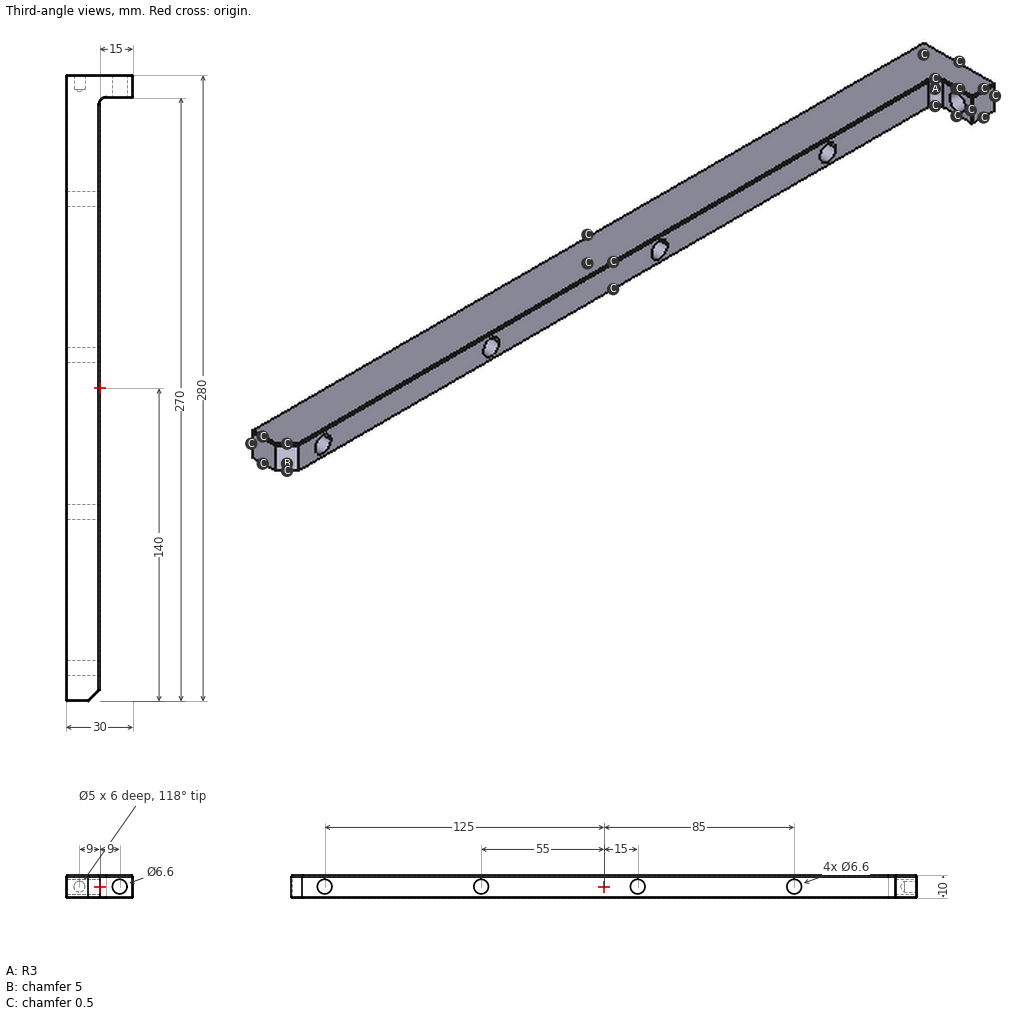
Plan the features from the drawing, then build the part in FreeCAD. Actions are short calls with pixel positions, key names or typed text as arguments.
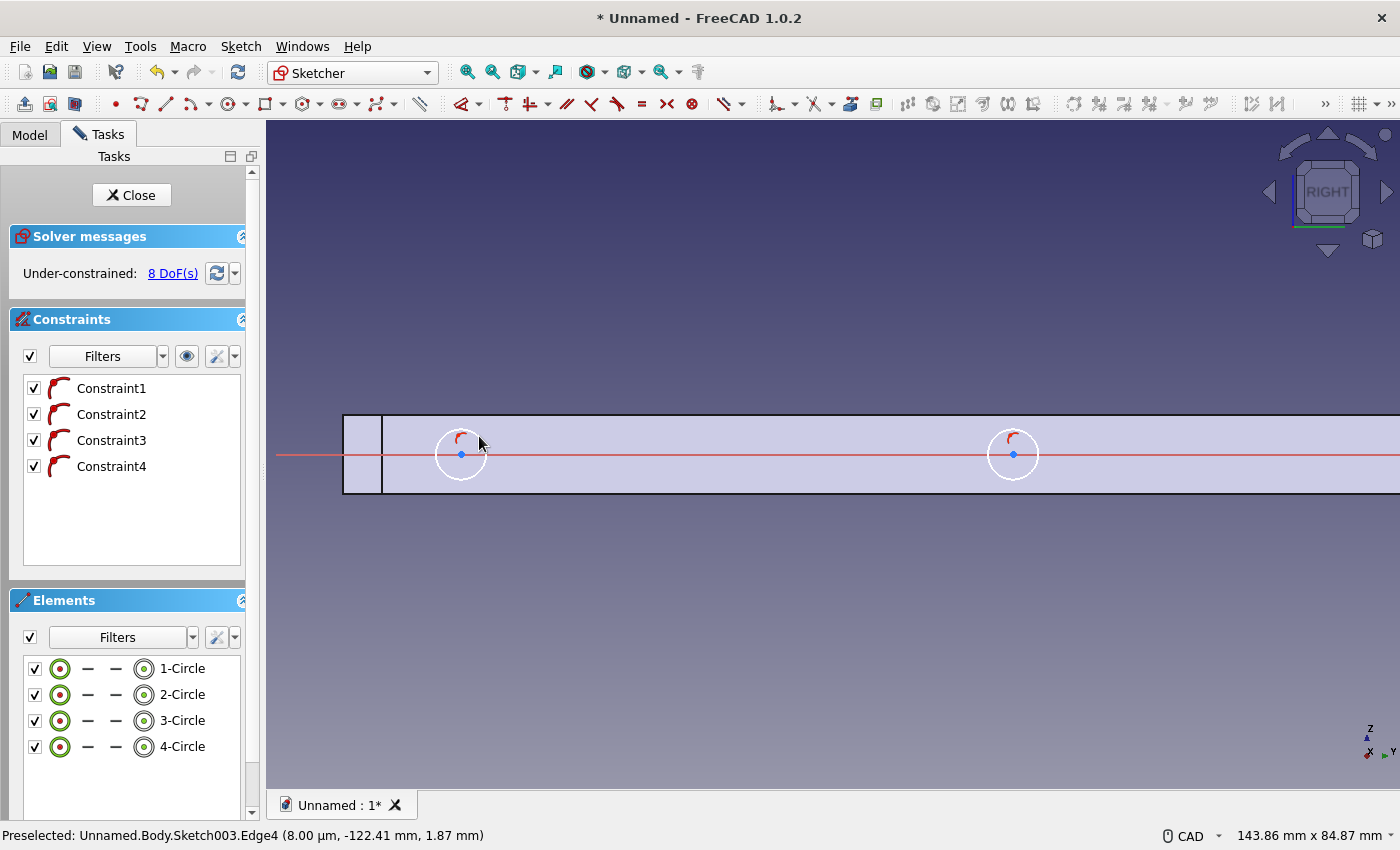
scroll(459, 455, down, 5)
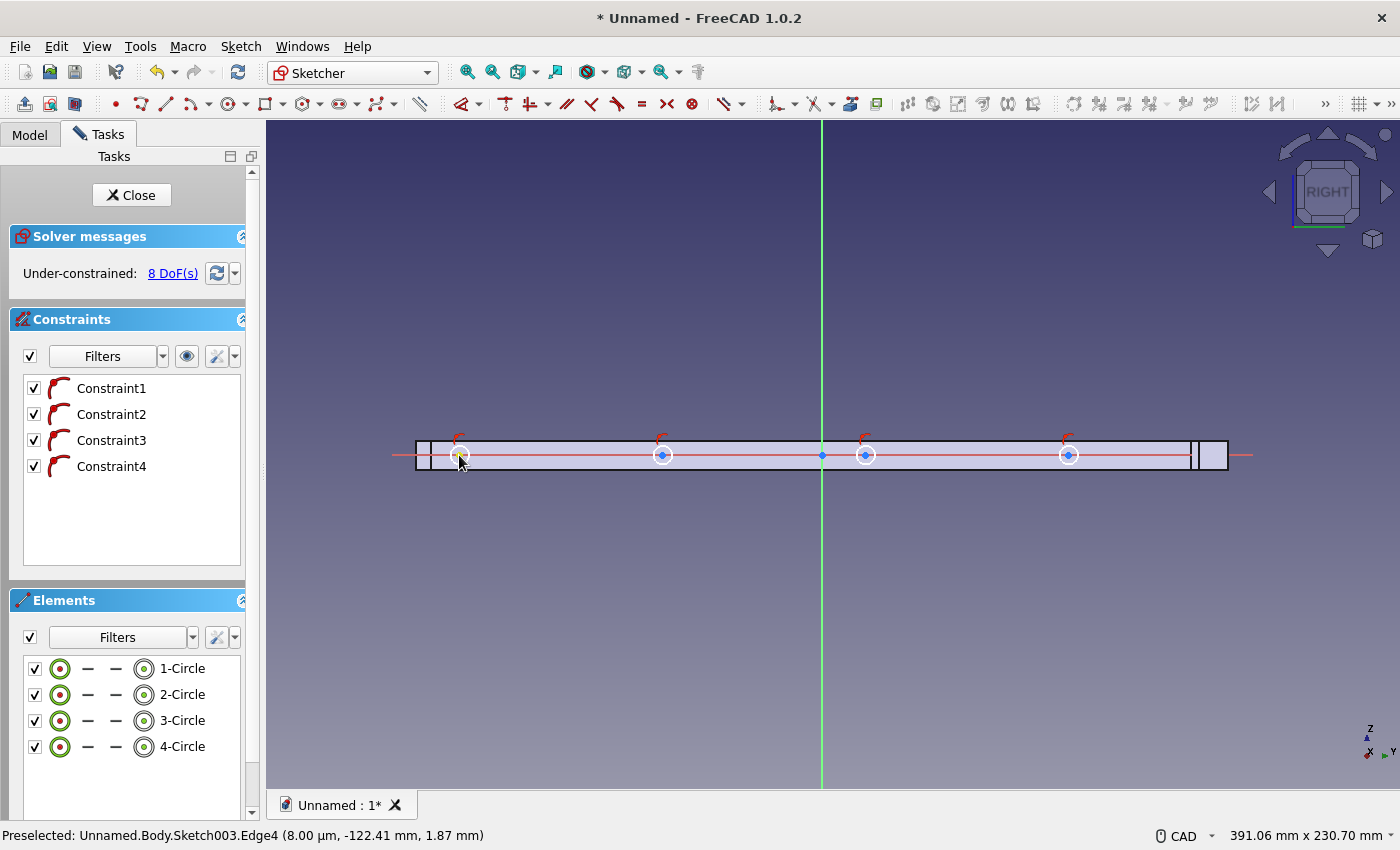
scroll(1075, 449, up, 4)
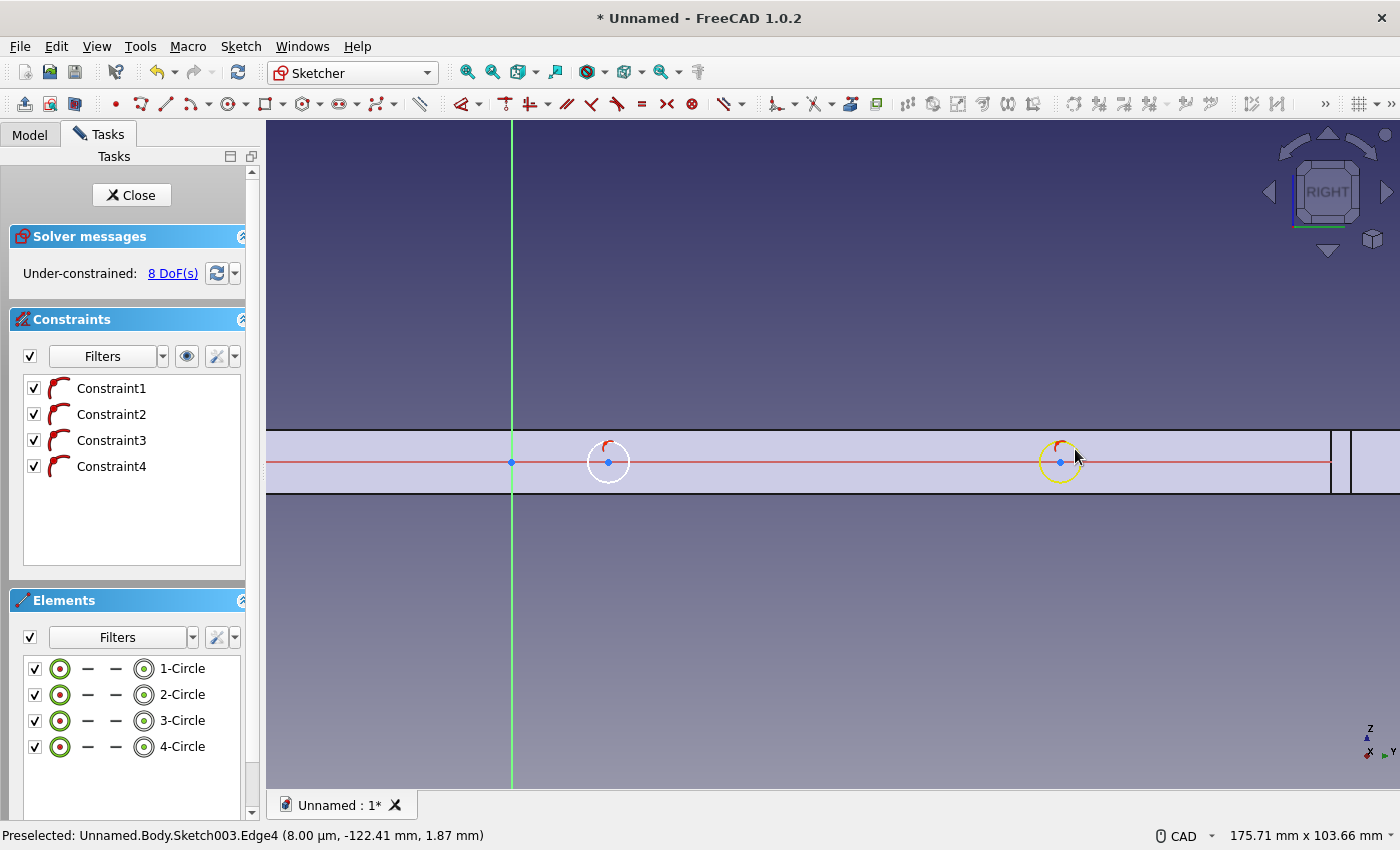
click(1075, 447)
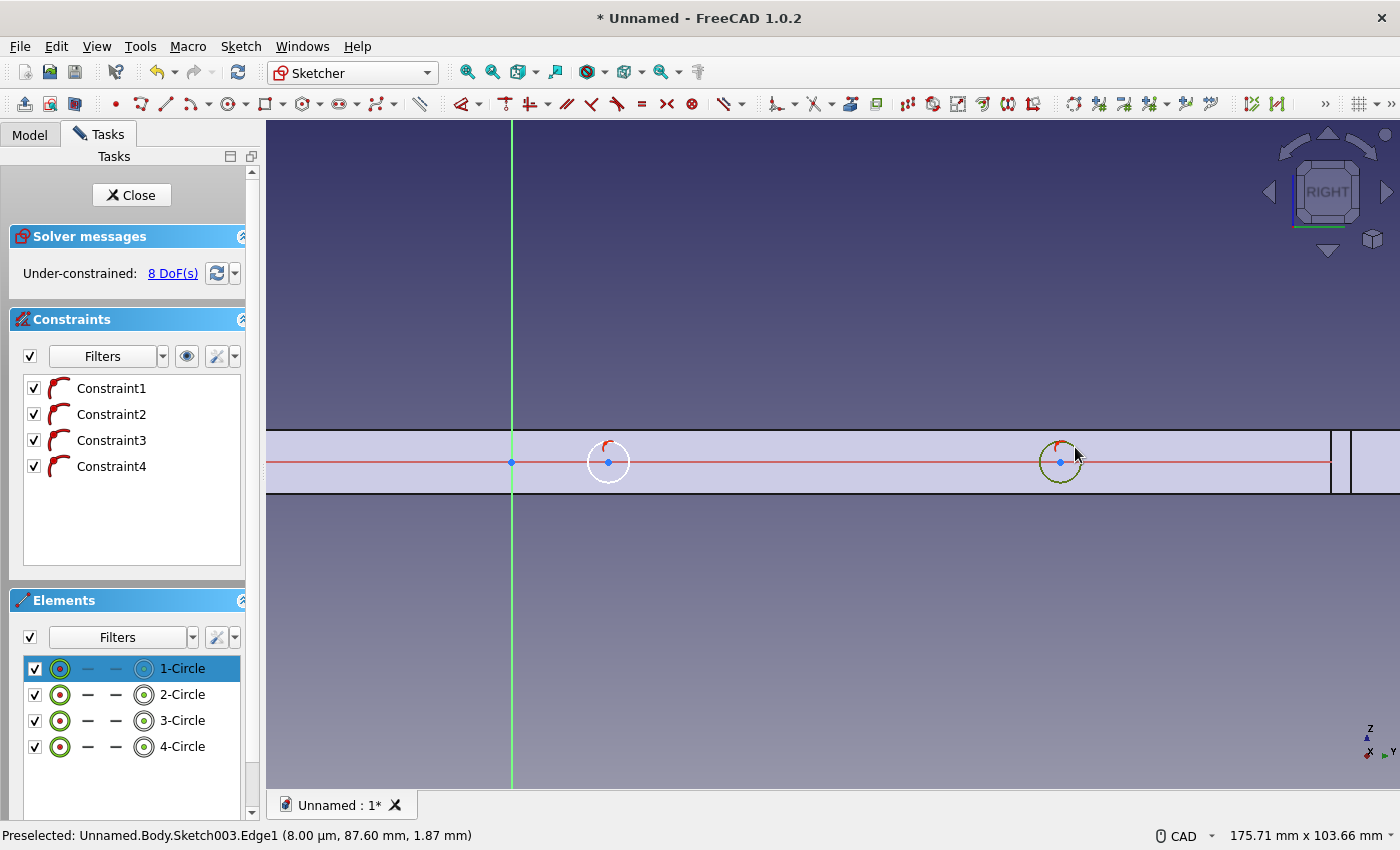
click(623, 447)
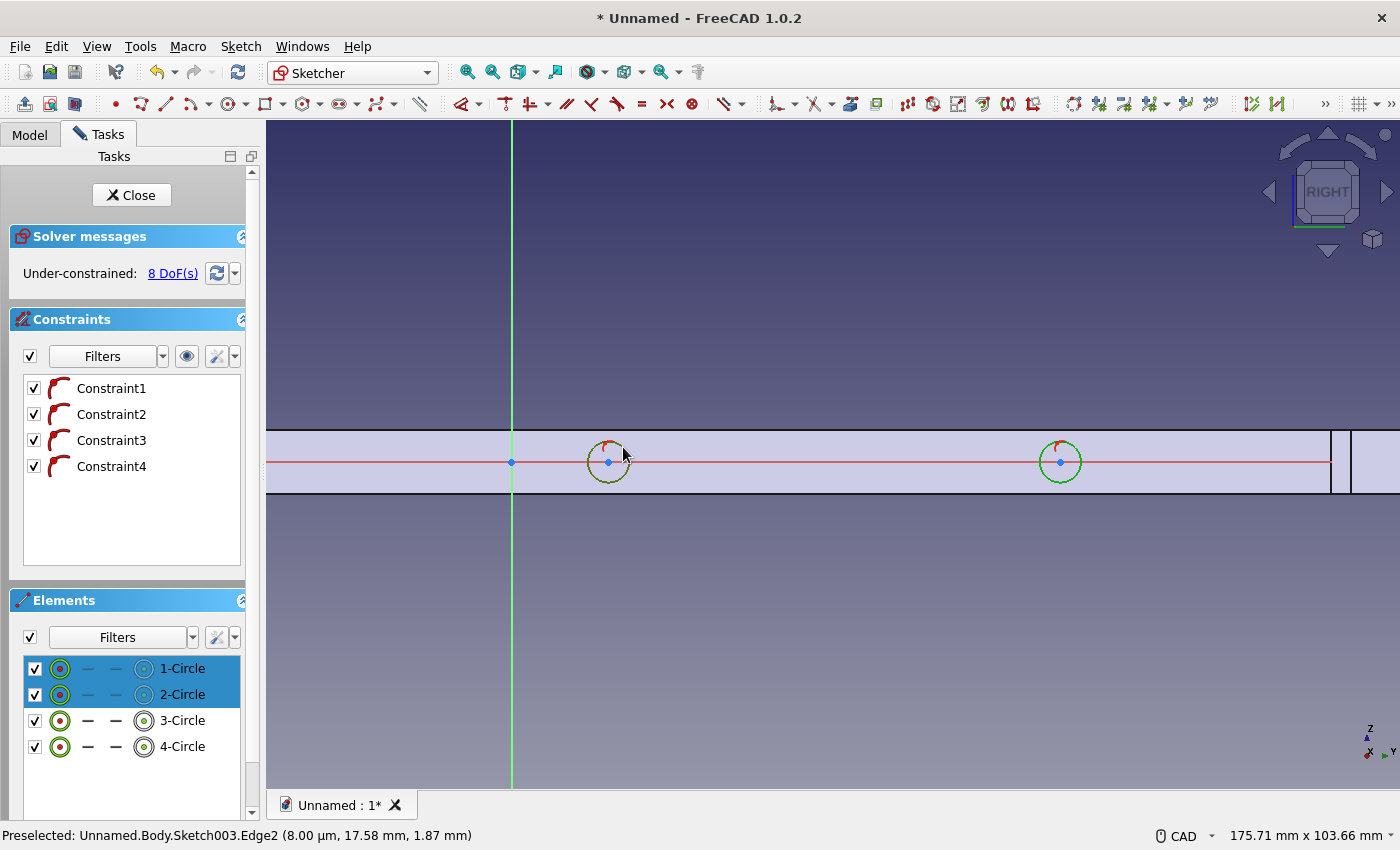
scroll(1076, 448, down, 4)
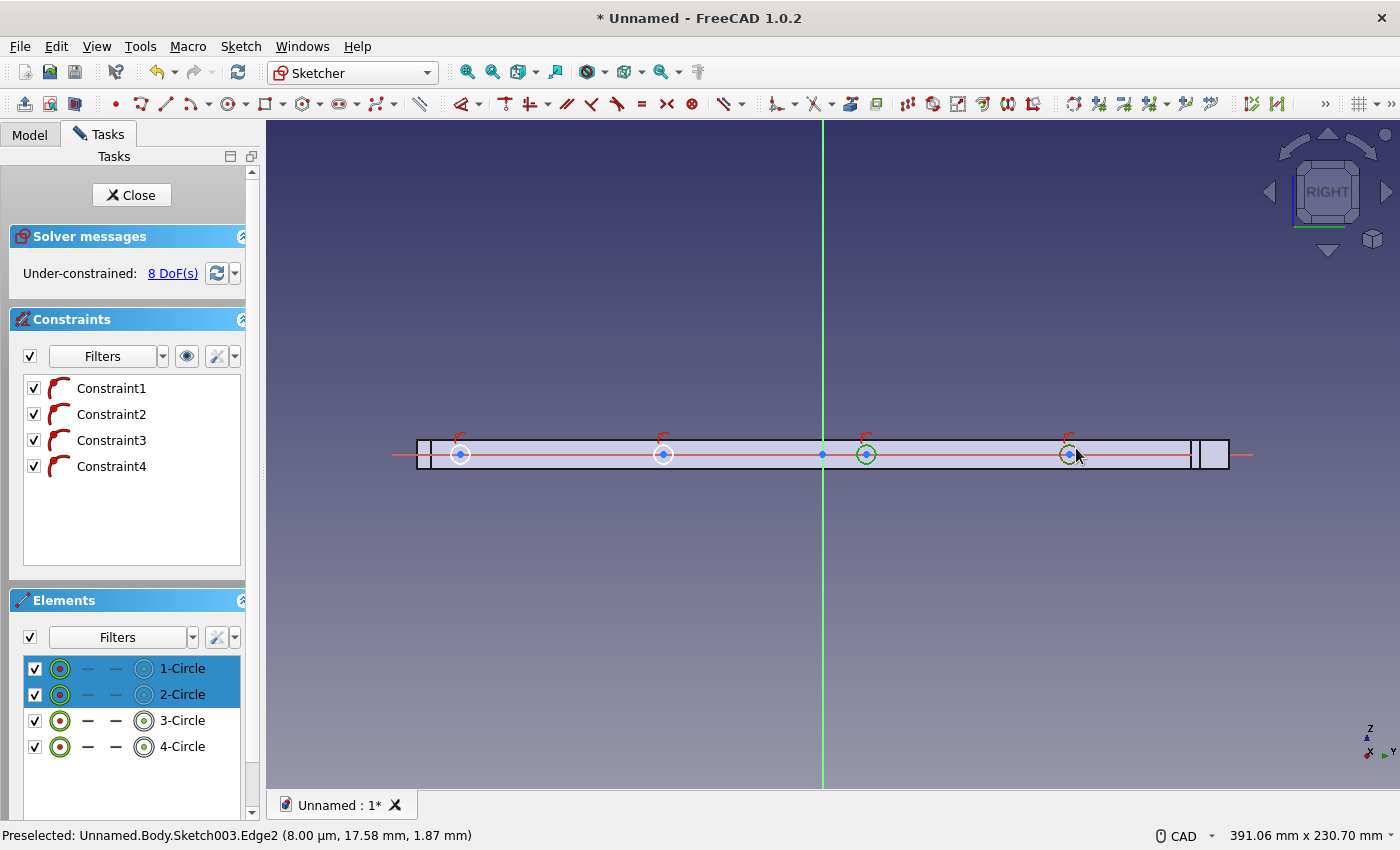
scroll(670, 448, up, 4)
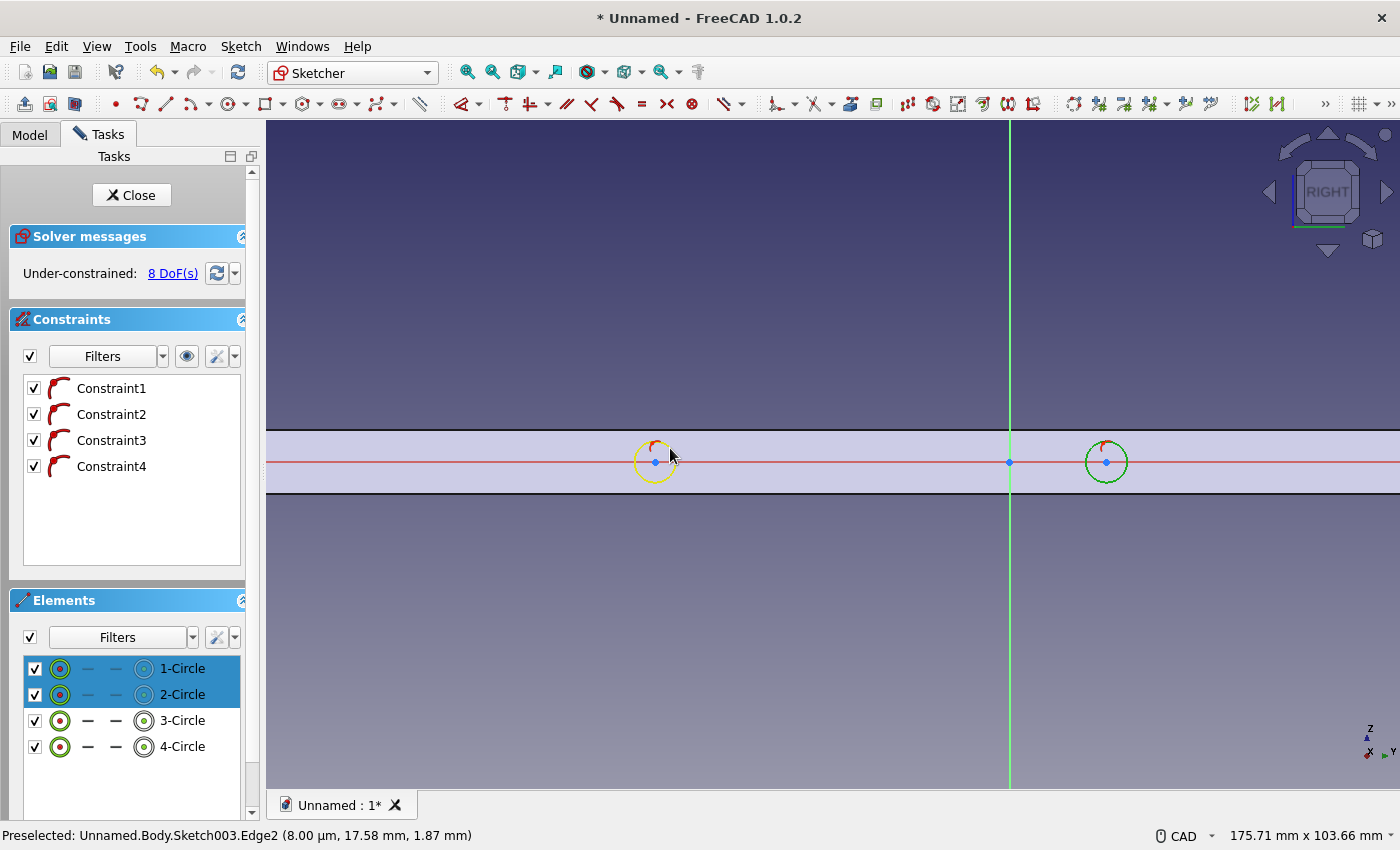
click(670, 447)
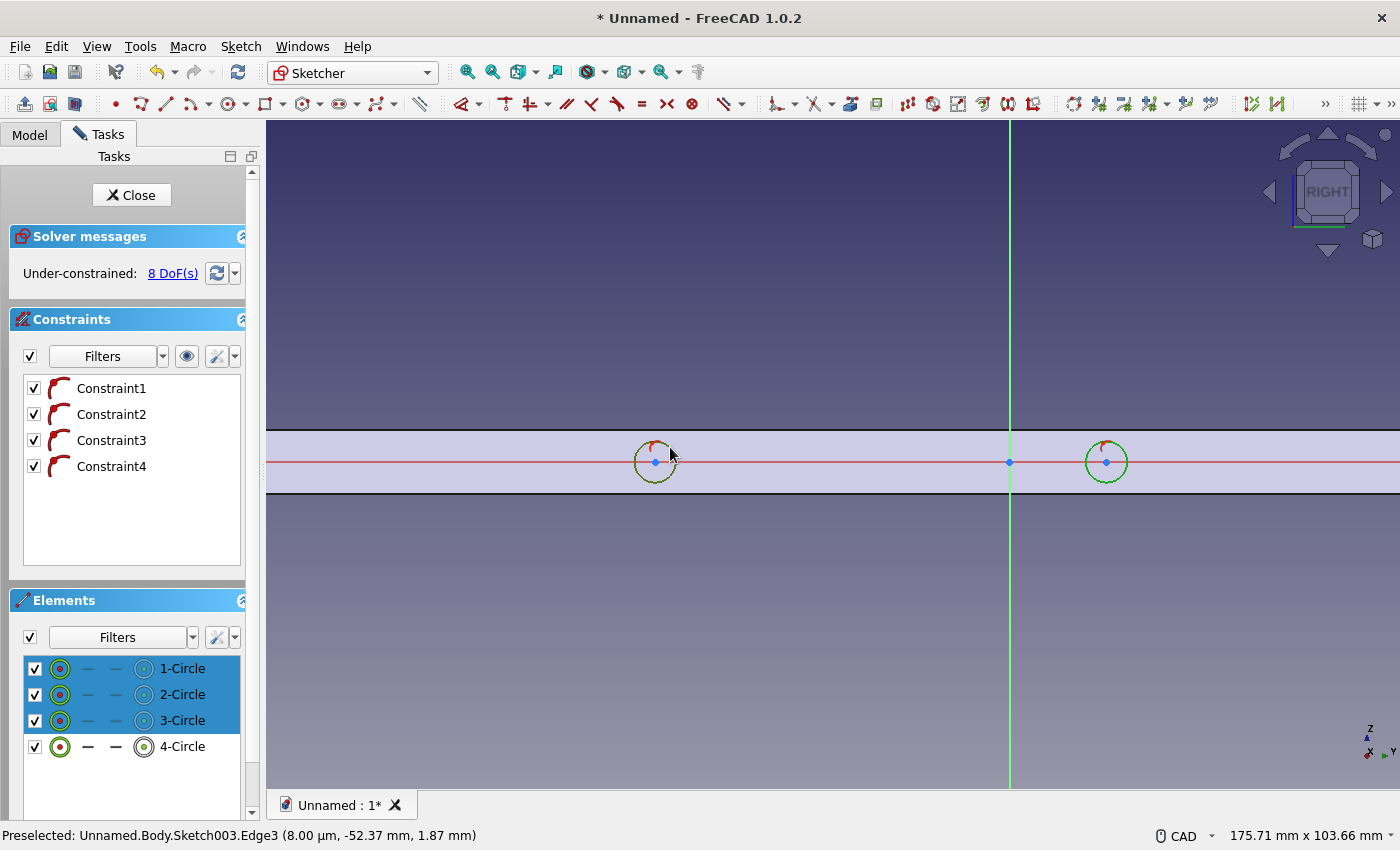
scroll(670, 448, down, 4)